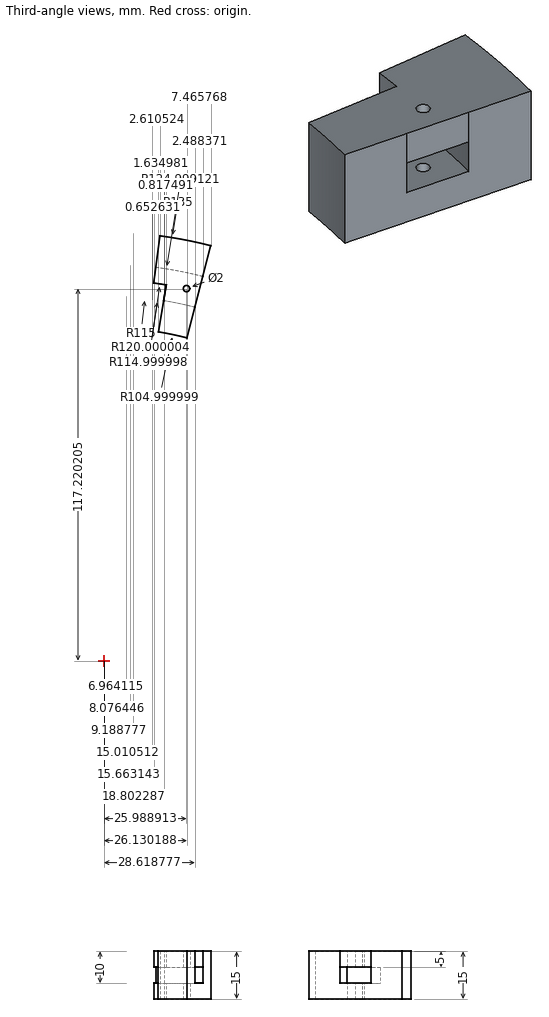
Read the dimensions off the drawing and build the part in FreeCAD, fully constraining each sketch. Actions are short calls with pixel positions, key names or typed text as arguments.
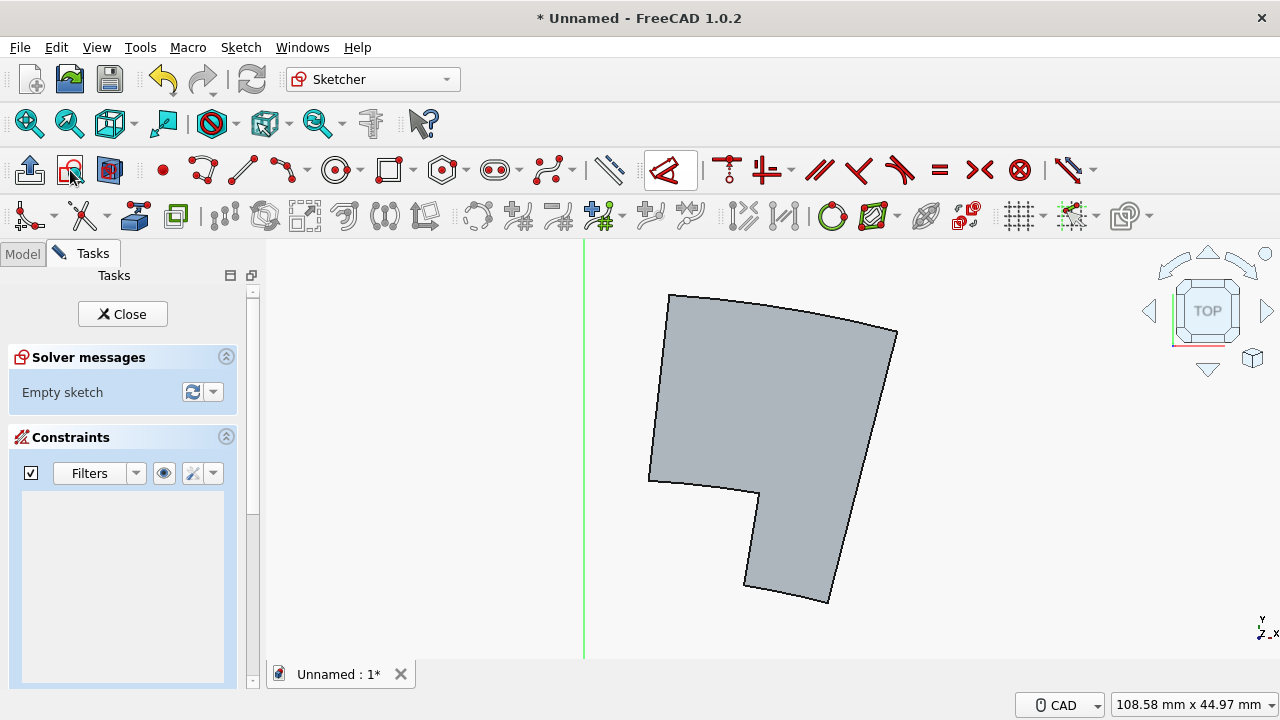
scroll(836, 459, up, 13)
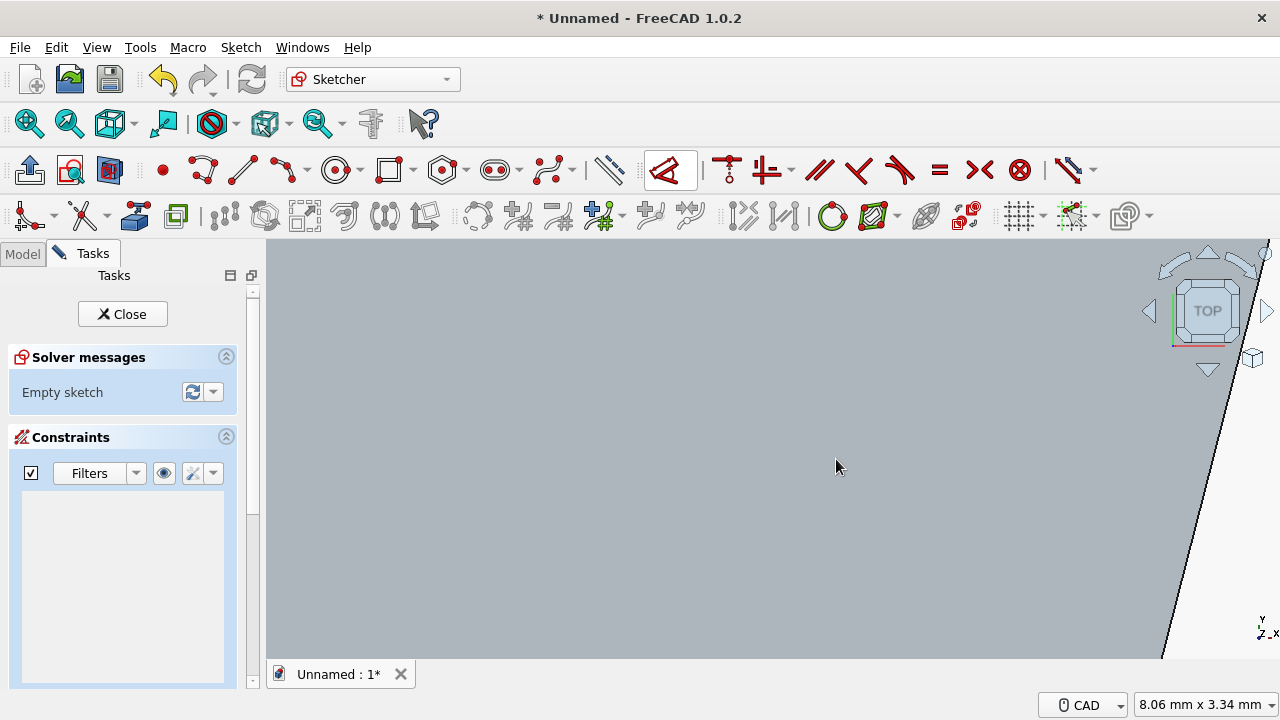
click(336, 170)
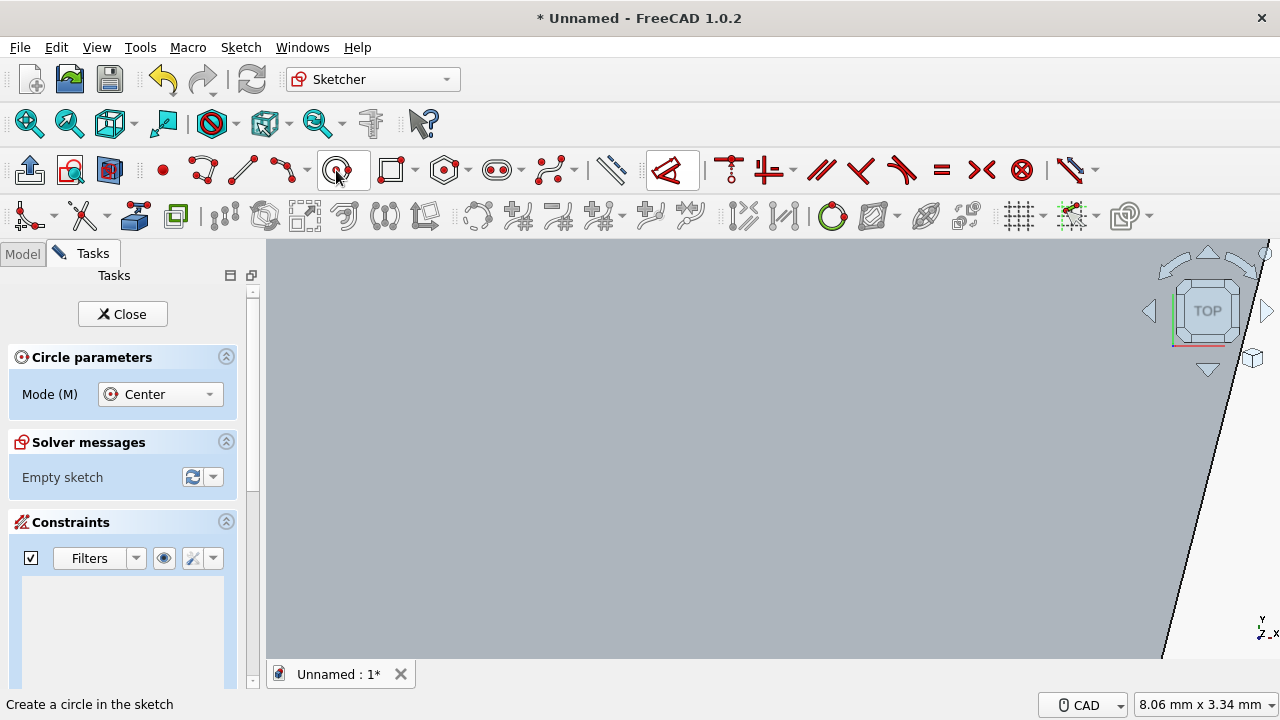
click(699, 440)
click(787, 351)
key(Escape)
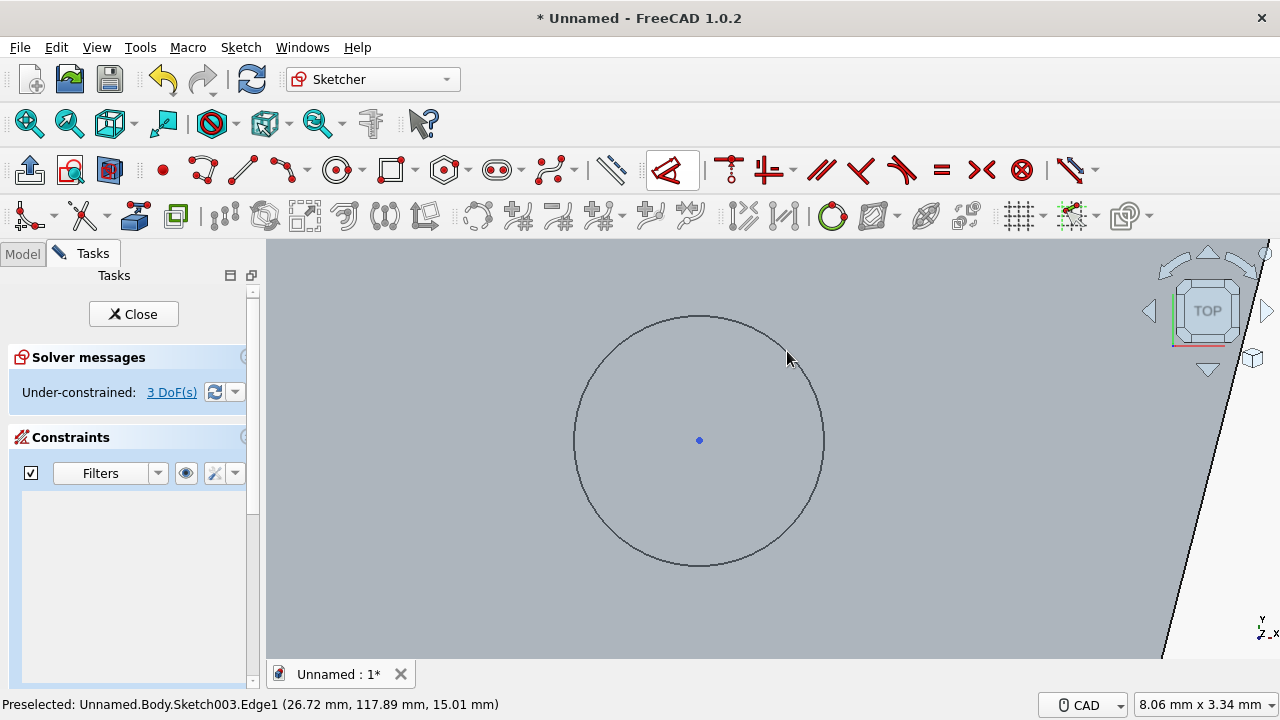
click(787, 352)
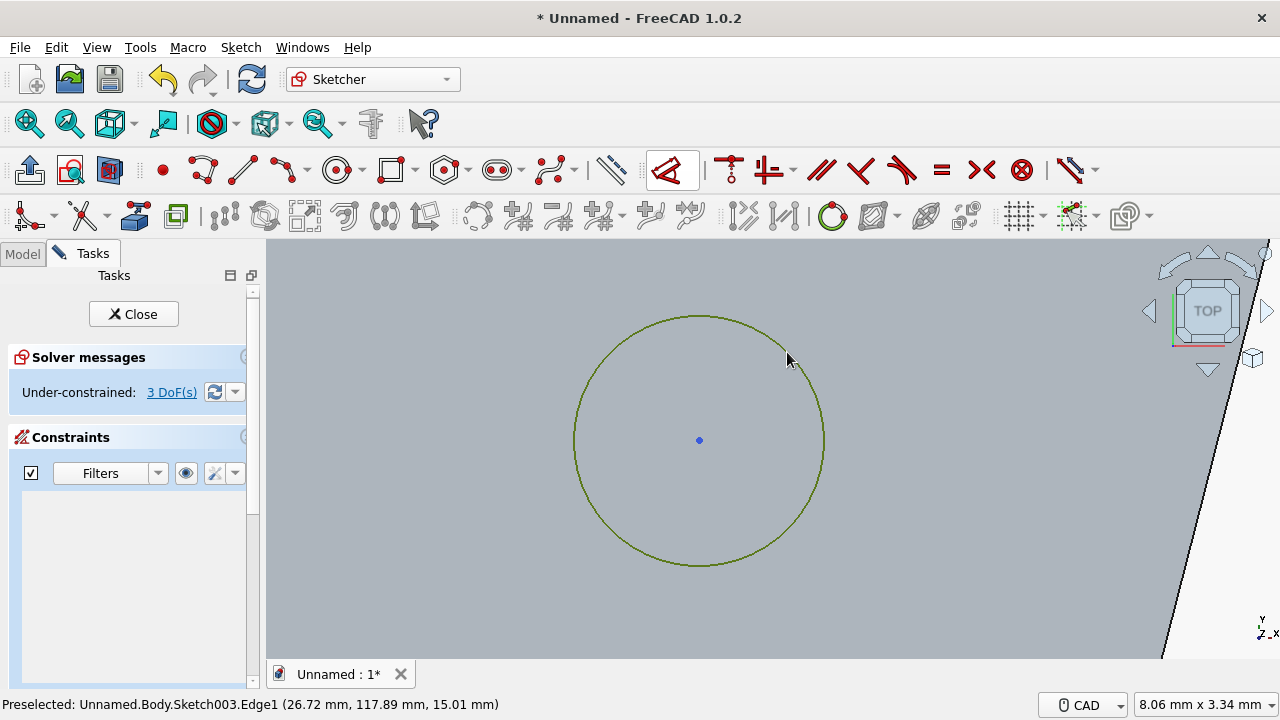
key(k)
key(o)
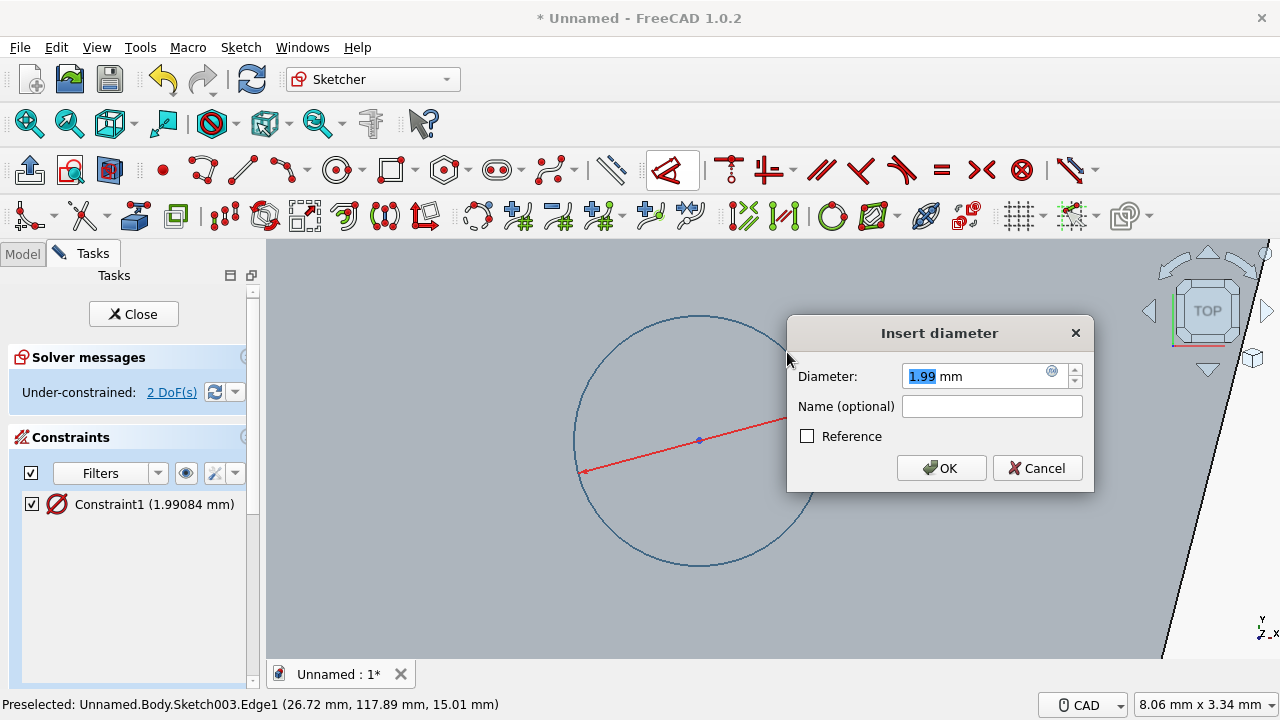
text(2)
key(Return)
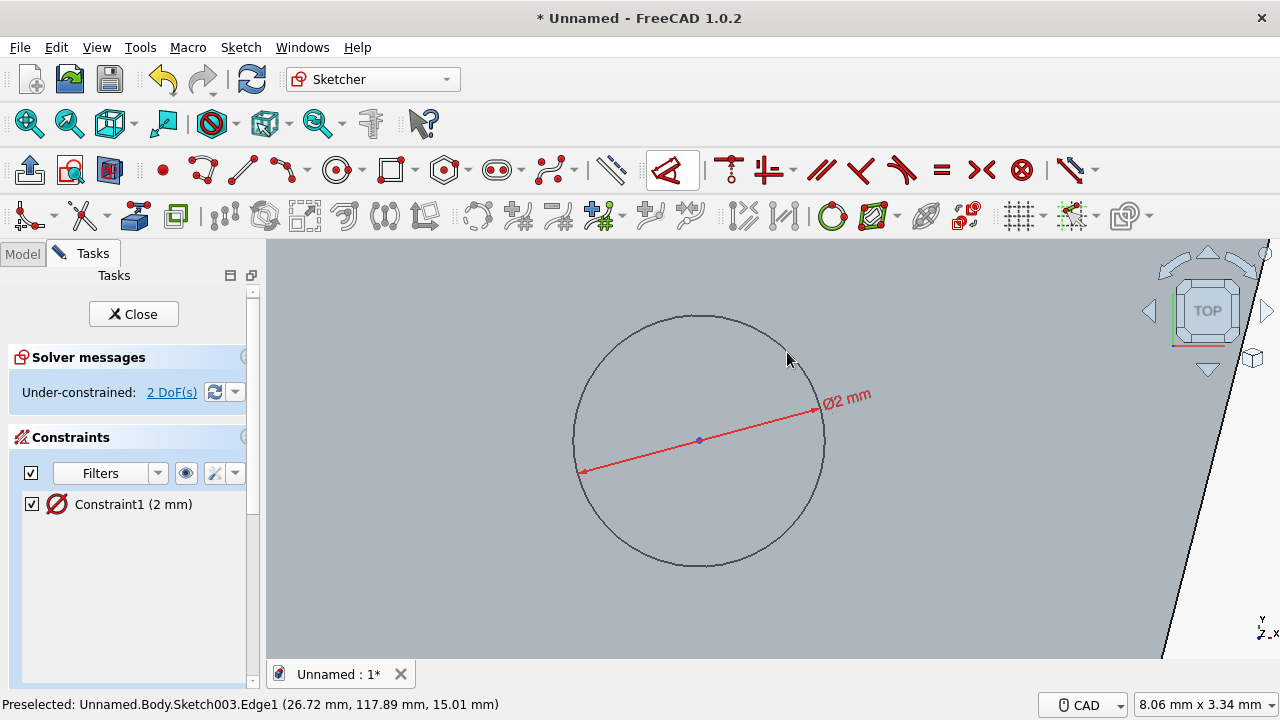
click(699, 441)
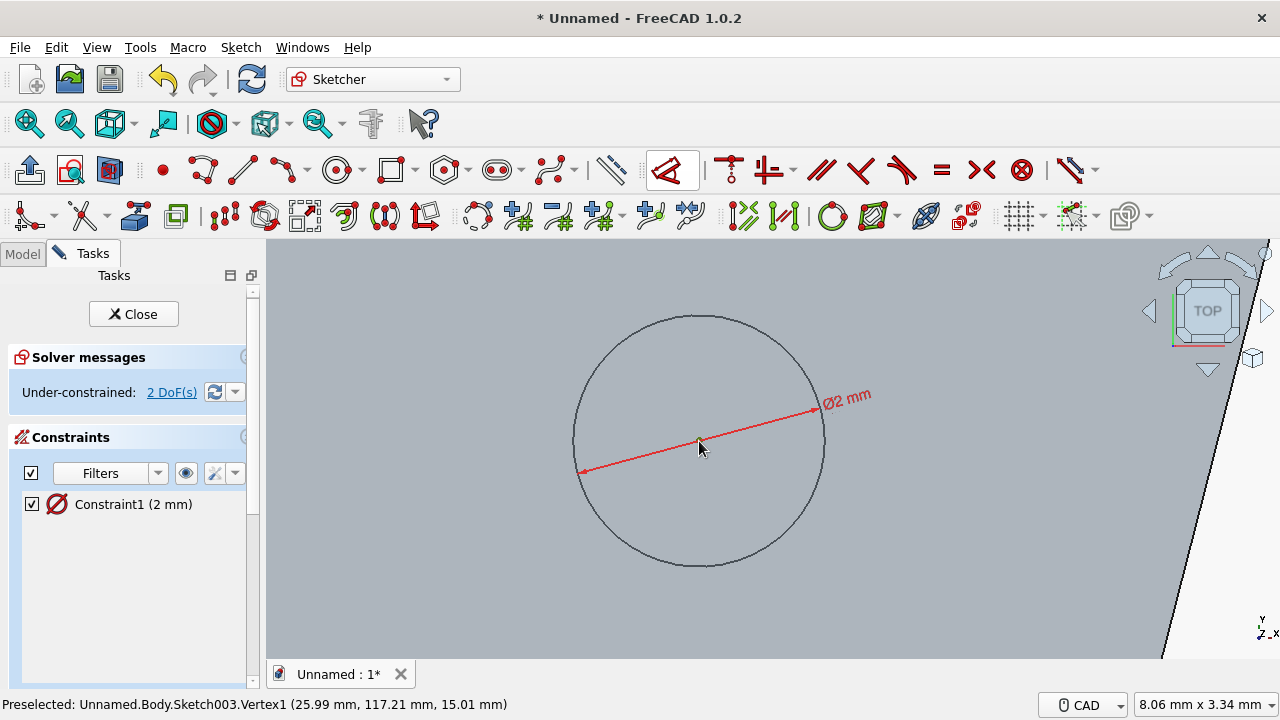
click(694, 170)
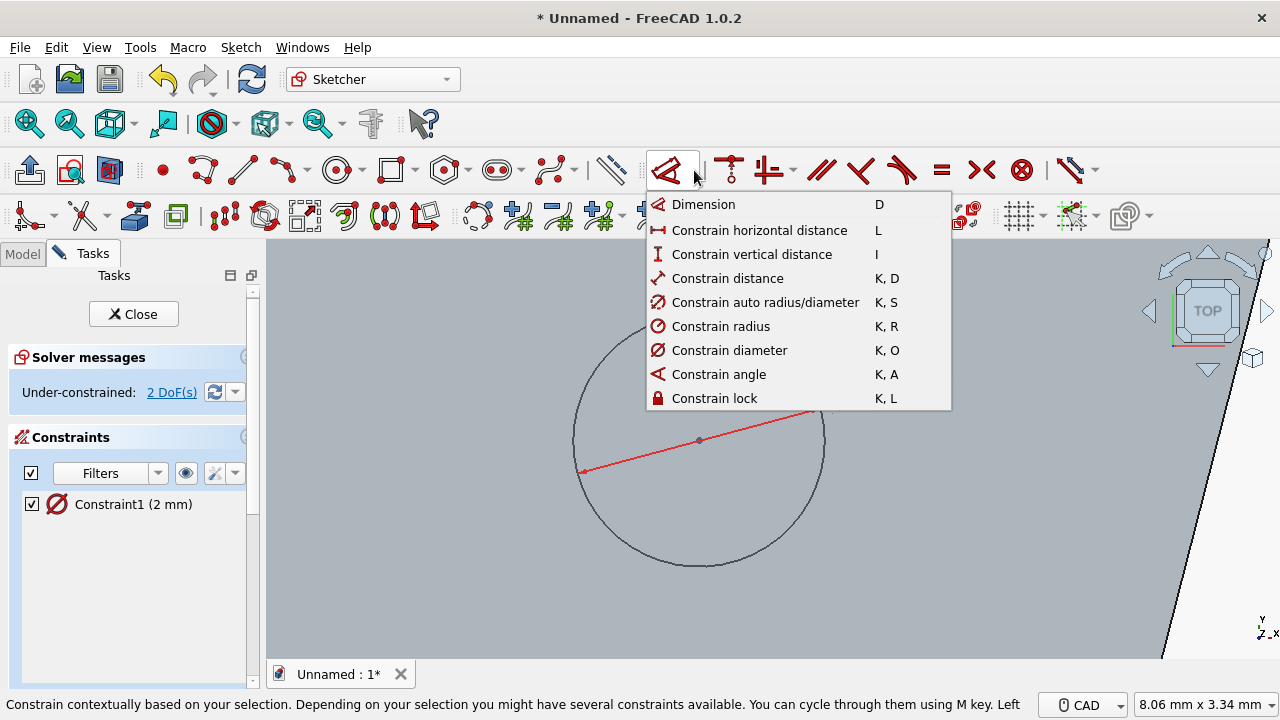
click(799, 230)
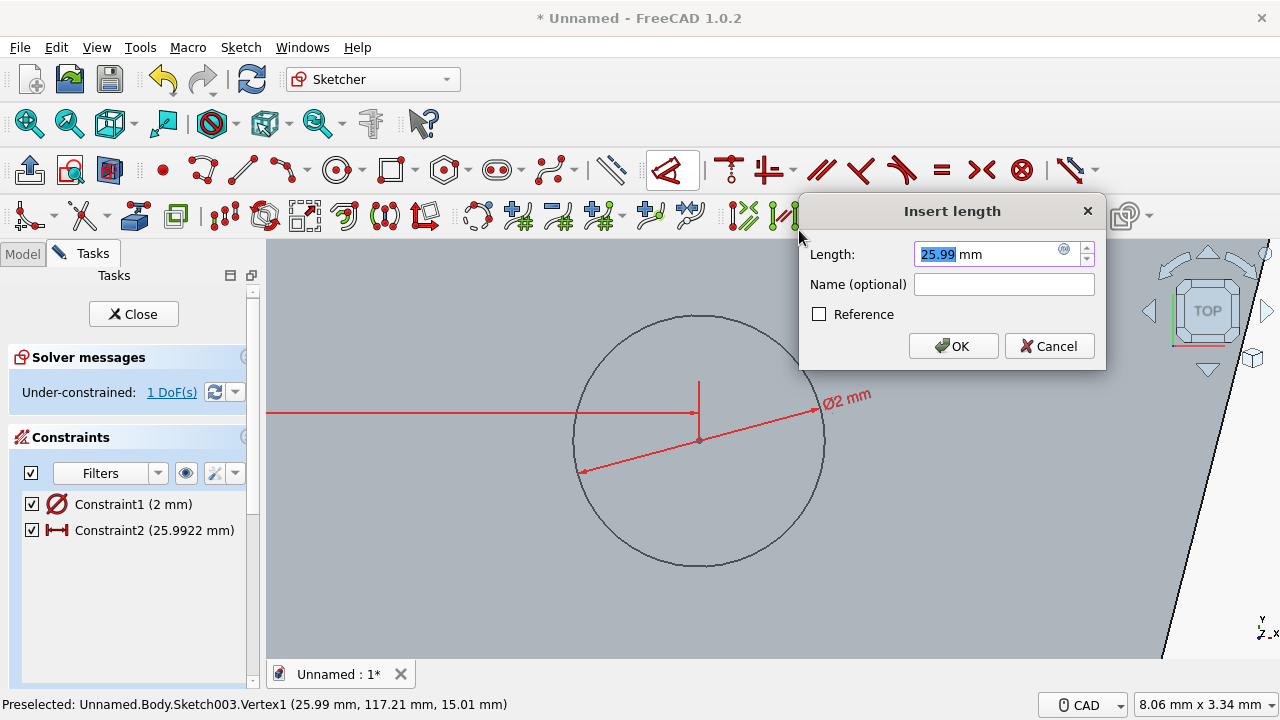
text(25.988913)
key(Return)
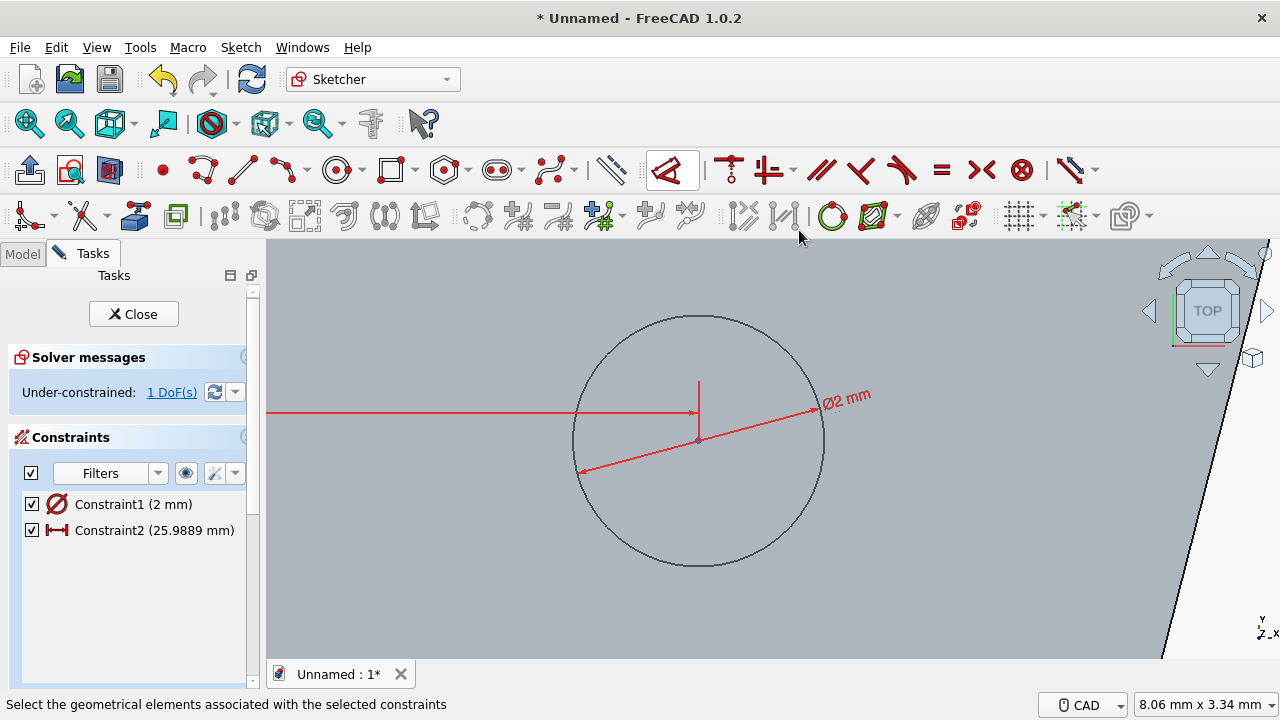
click(699, 441)